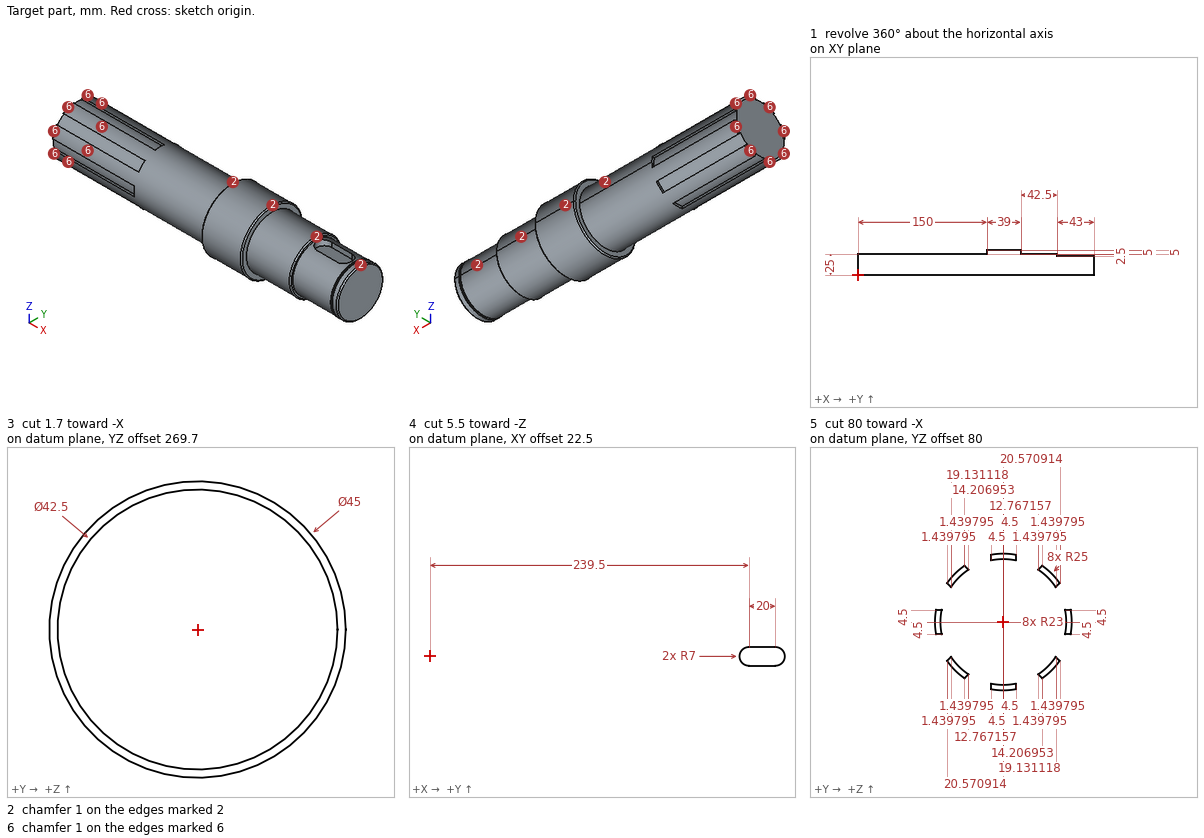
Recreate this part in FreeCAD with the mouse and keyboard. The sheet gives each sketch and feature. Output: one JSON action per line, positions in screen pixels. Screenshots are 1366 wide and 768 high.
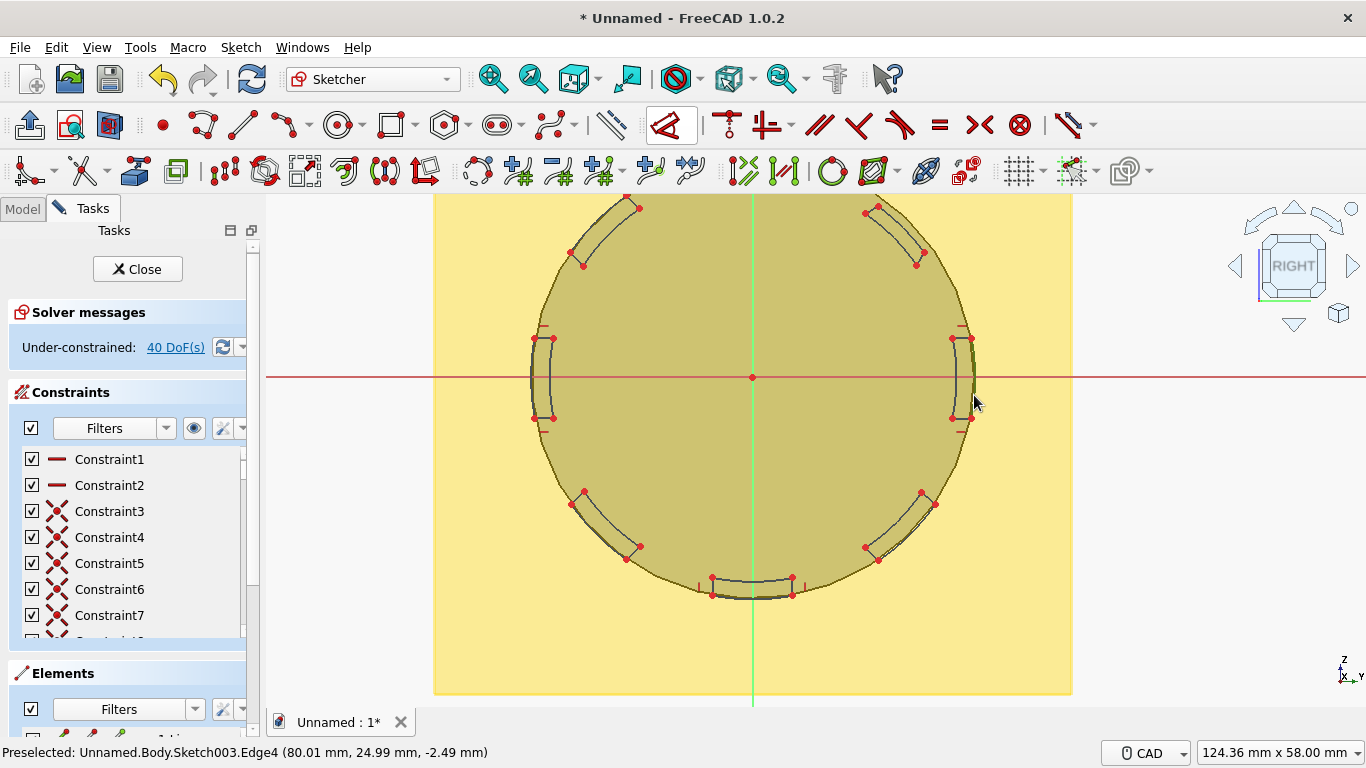
{"action": "left_click", "coordinate": [912, 237]}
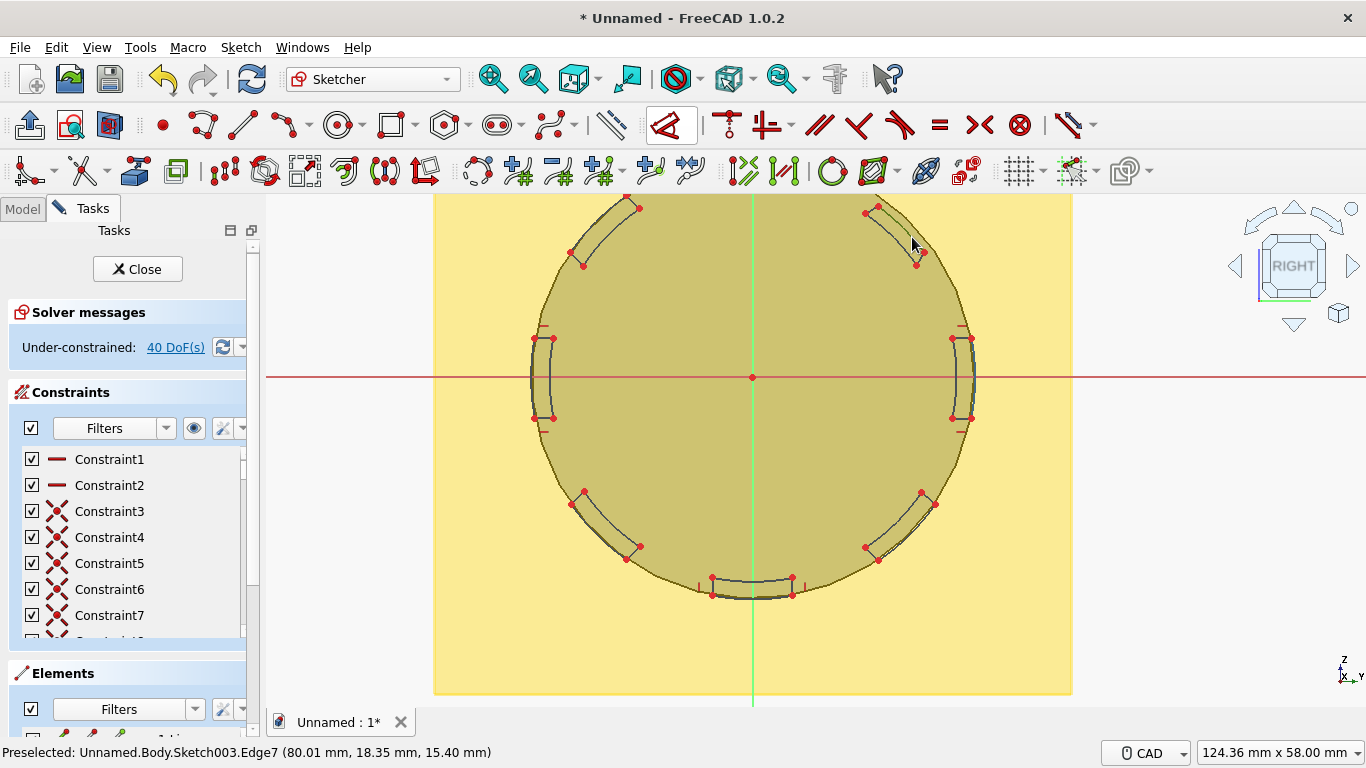
{"action": "scroll", "coordinate": [737, 599], "scroll_direction": "down", "scroll_amount": 2}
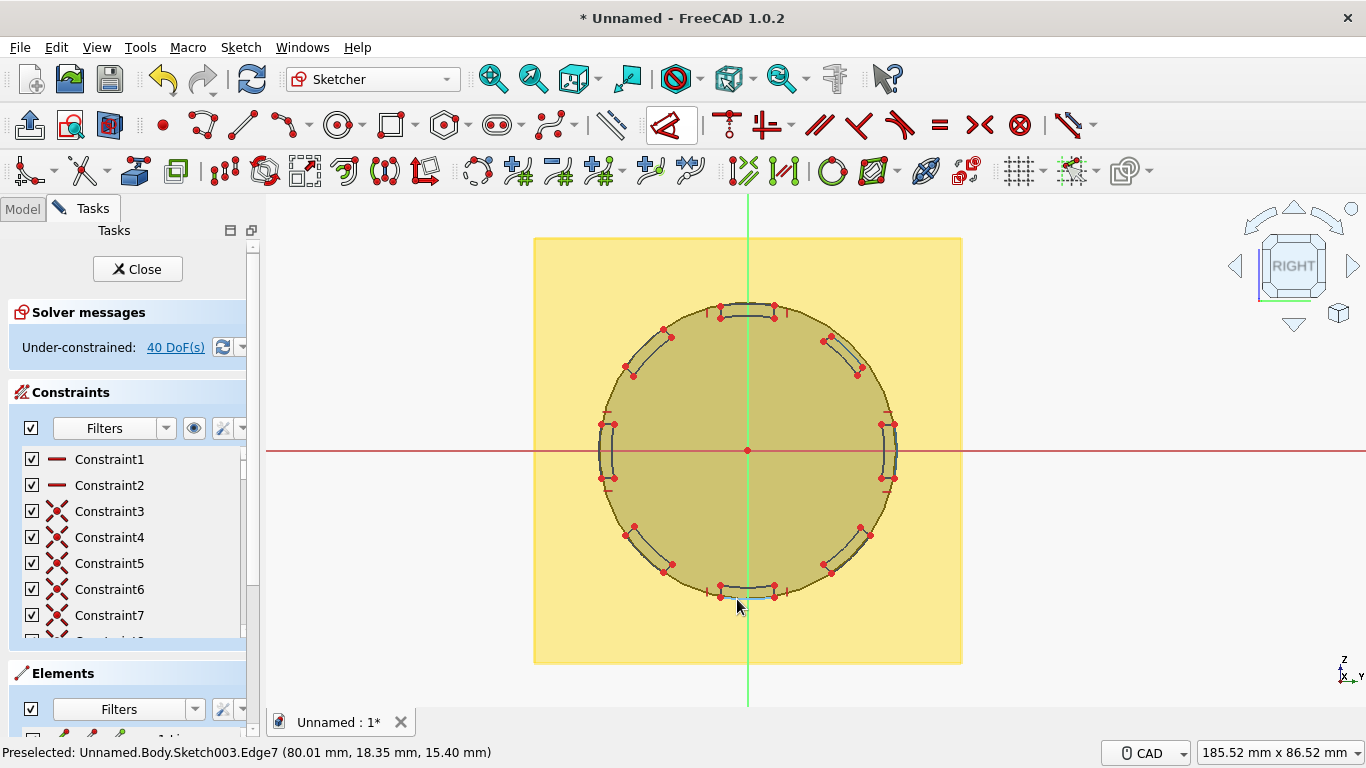
{"action": "scroll", "coordinate": [758, 304], "scroll_direction": "up", "scroll_amount": 2}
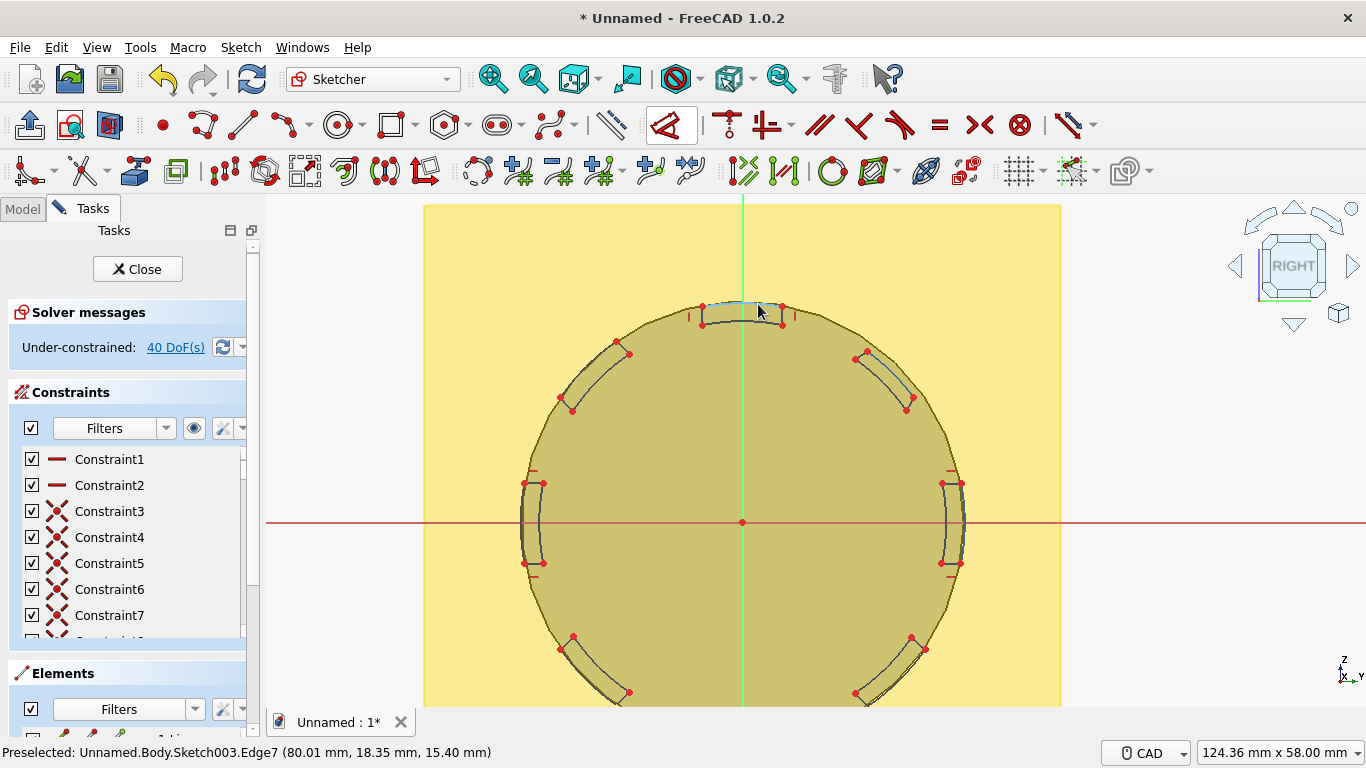
{"action": "left_click", "coordinate": [758, 304]}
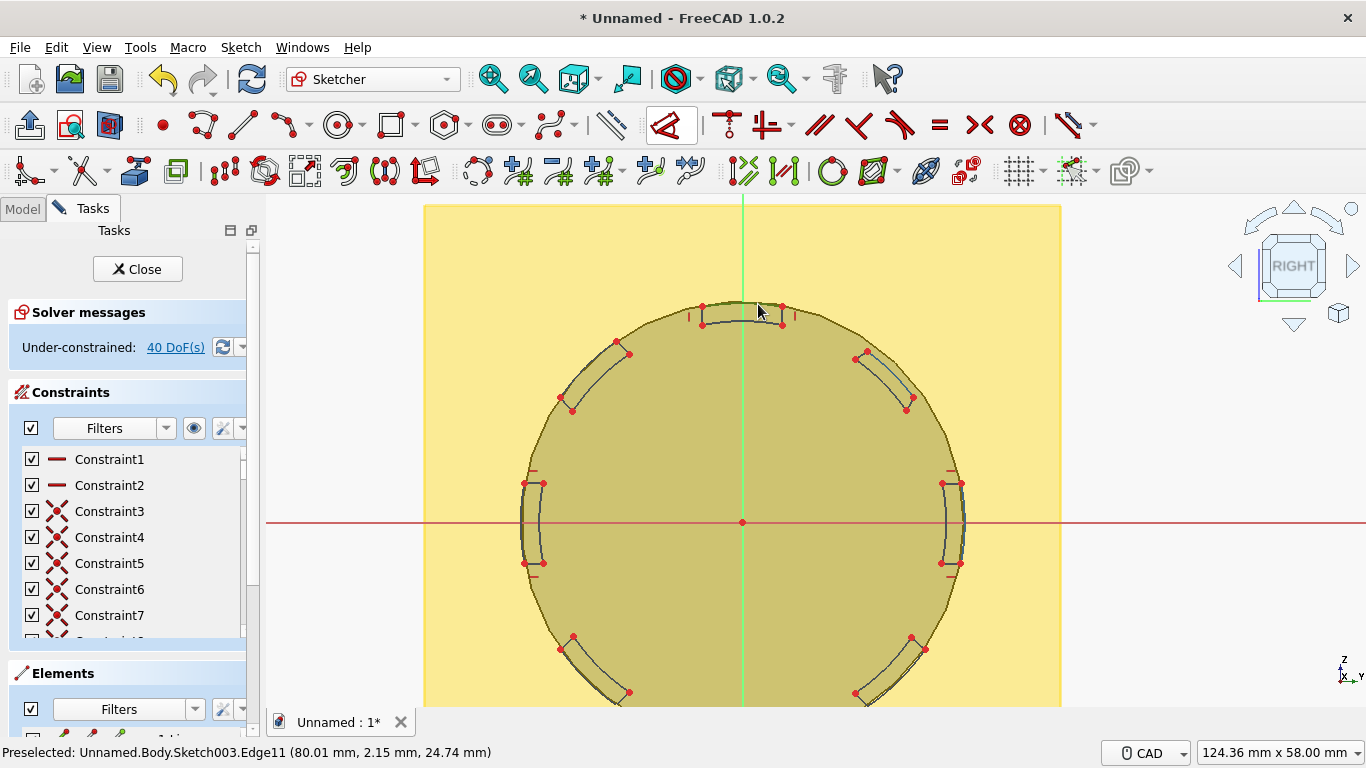
{"action": "left_click", "coordinate": [597, 356]}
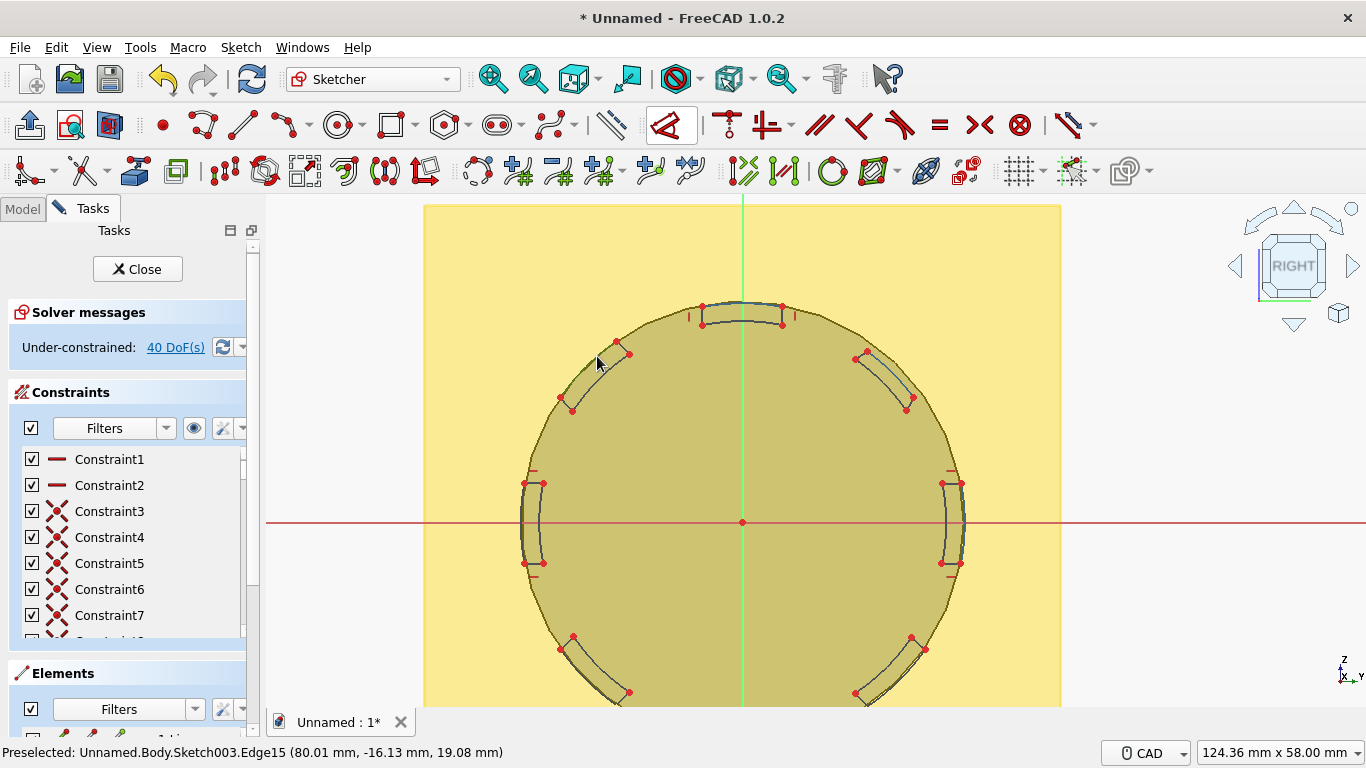
{"action": "left_click", "coordinate": [521, 507]}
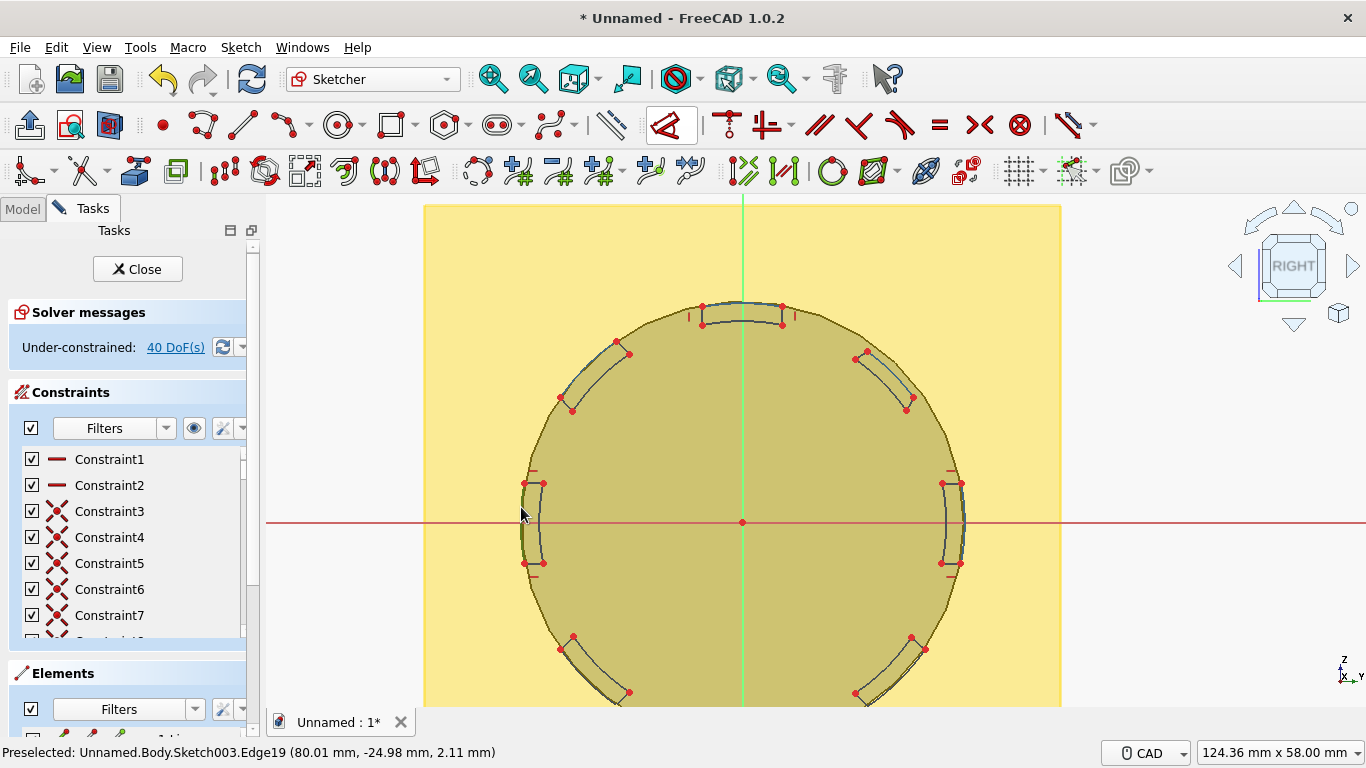
{"action": "left_click", "coordinate": [575, 668]}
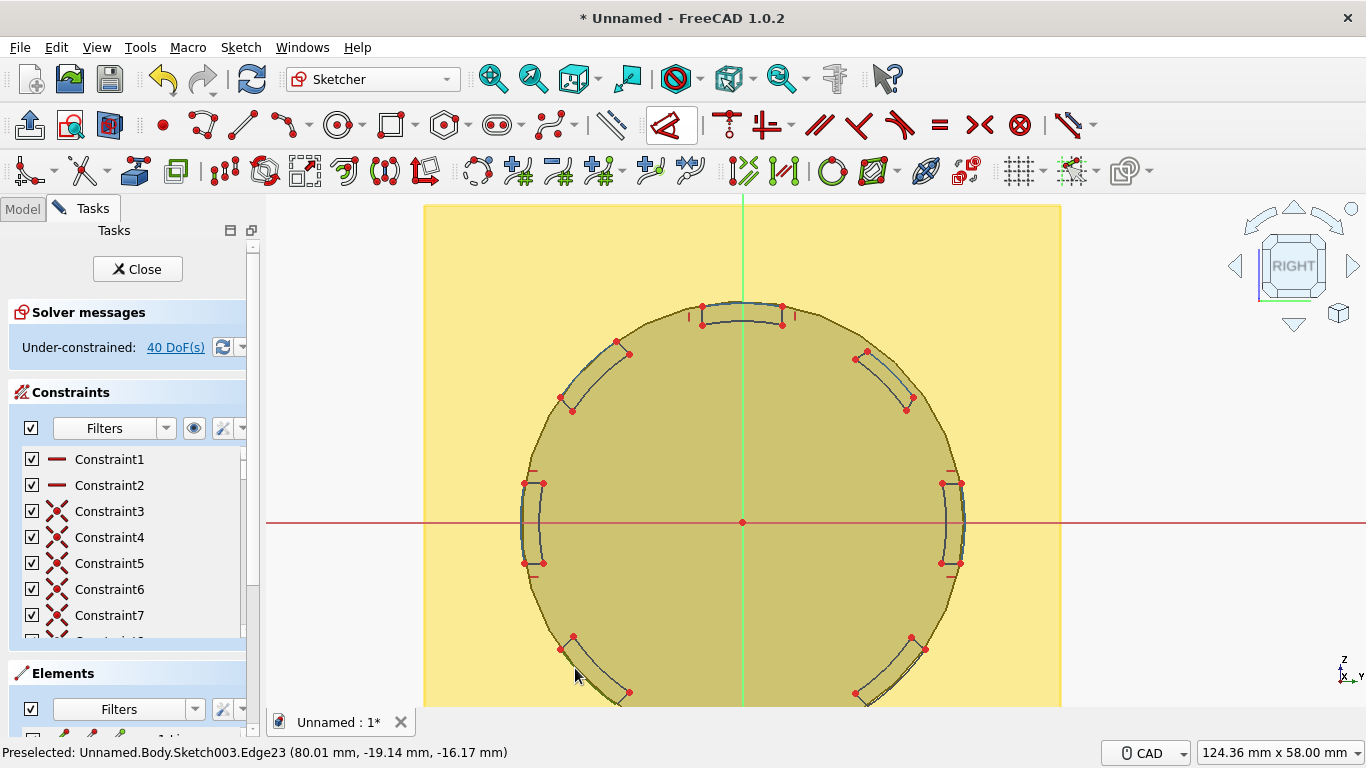
{"action": "scroll", "coordinate": [758, 303], "scroll_direction": "down", "scroll_amount": 2}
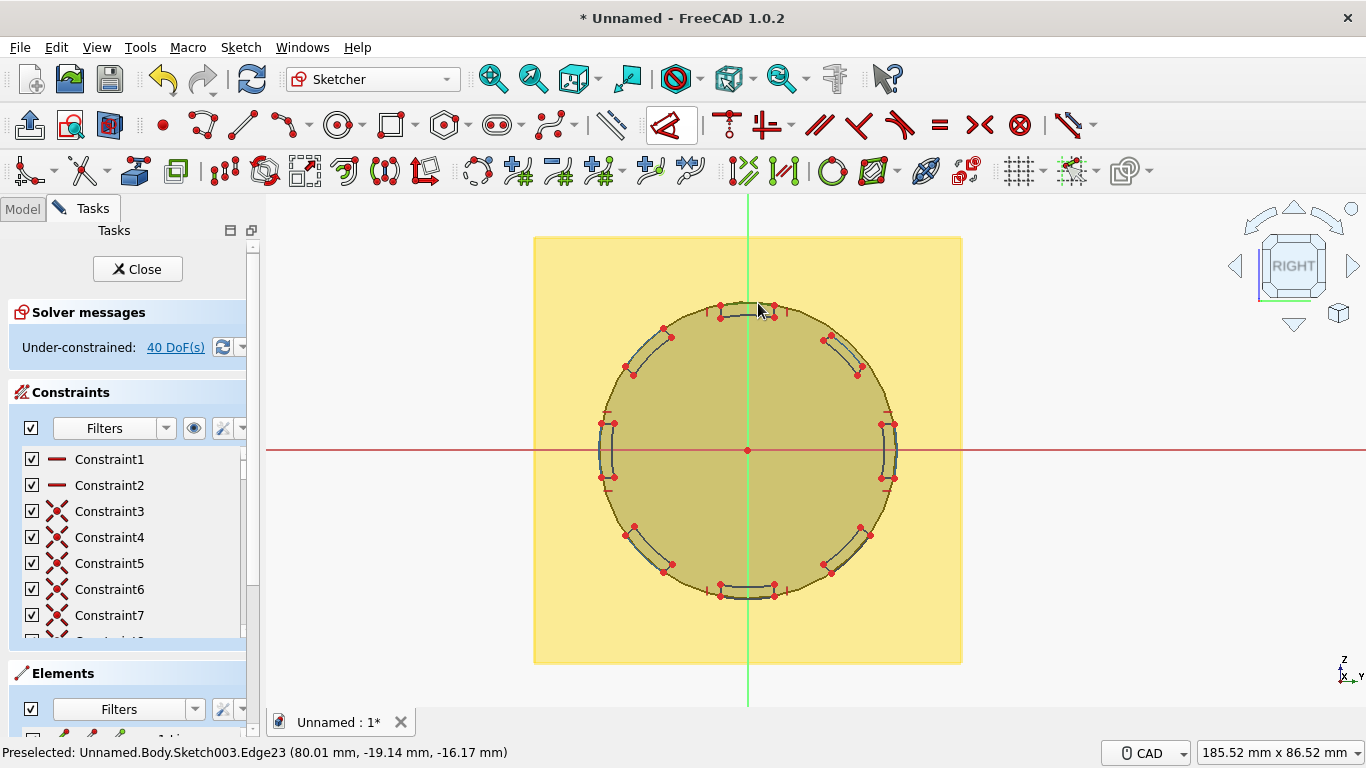
{"action": "scroll", "coordinate": [737, 599], "scroll_direction": "up", "scroll_amount": 2}